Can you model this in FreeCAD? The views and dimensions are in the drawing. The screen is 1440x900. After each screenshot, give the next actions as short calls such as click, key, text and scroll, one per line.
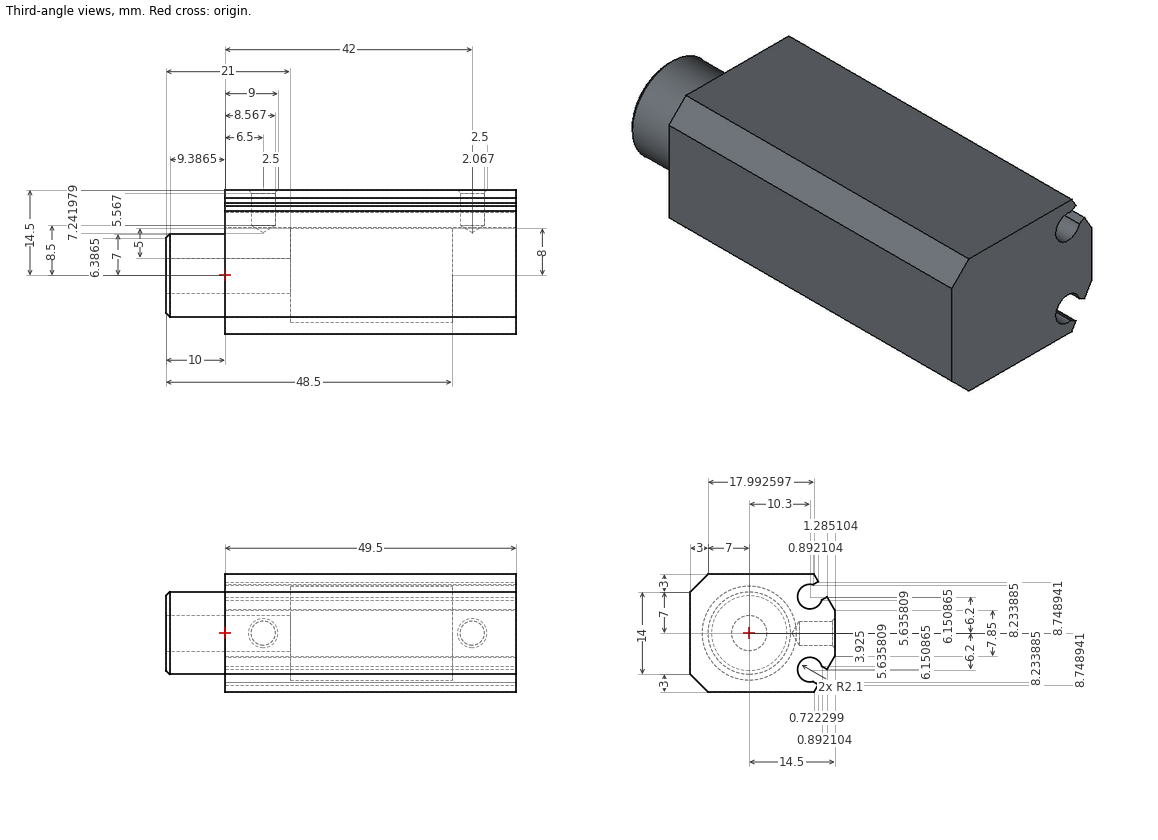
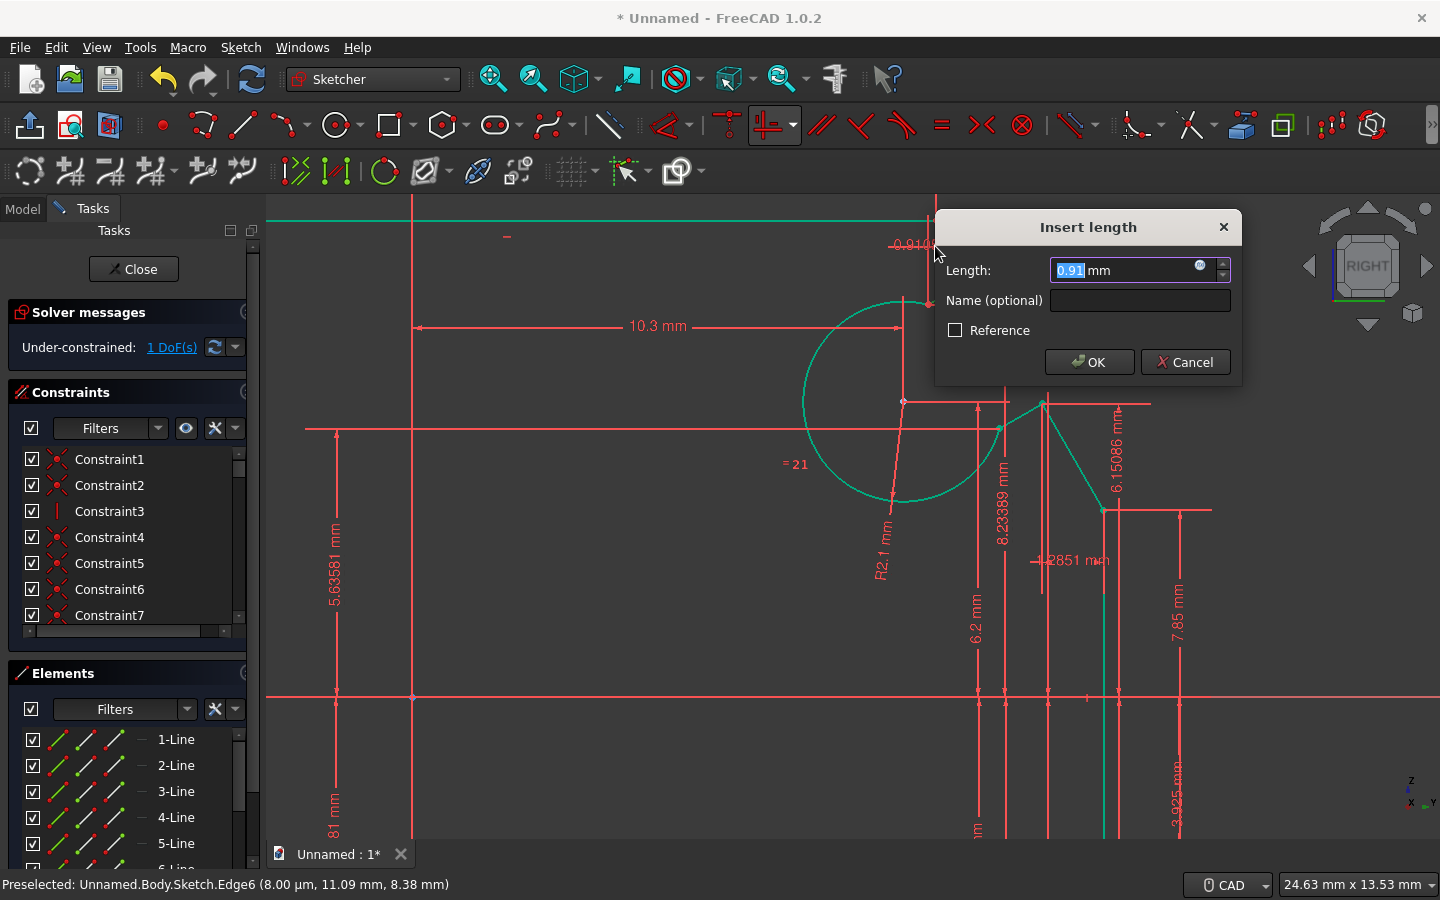
text(0.892104)
key(Return)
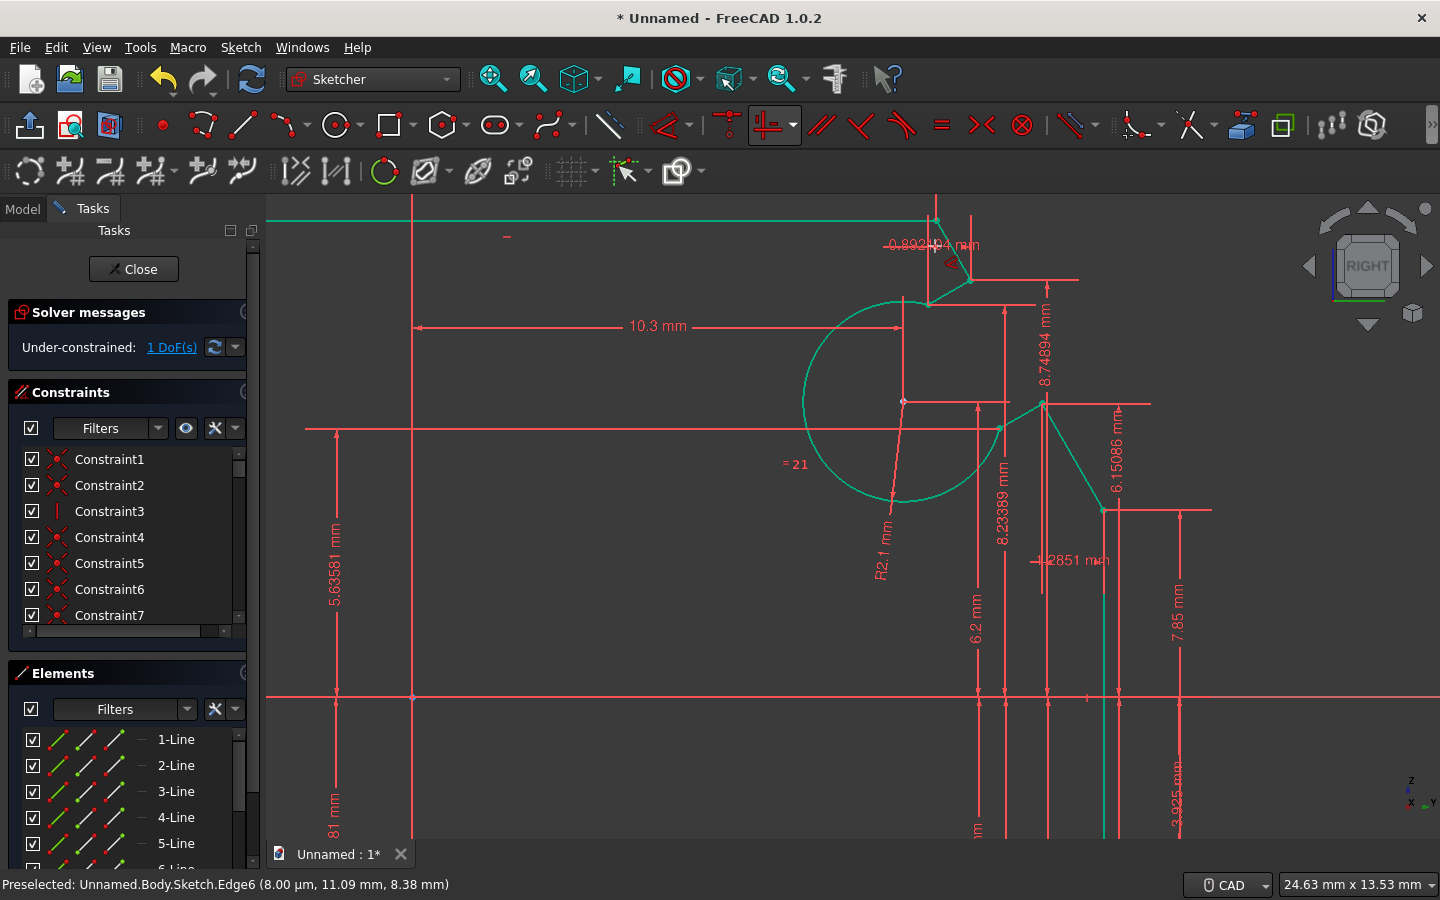
scroll(1001, 369, down, 4)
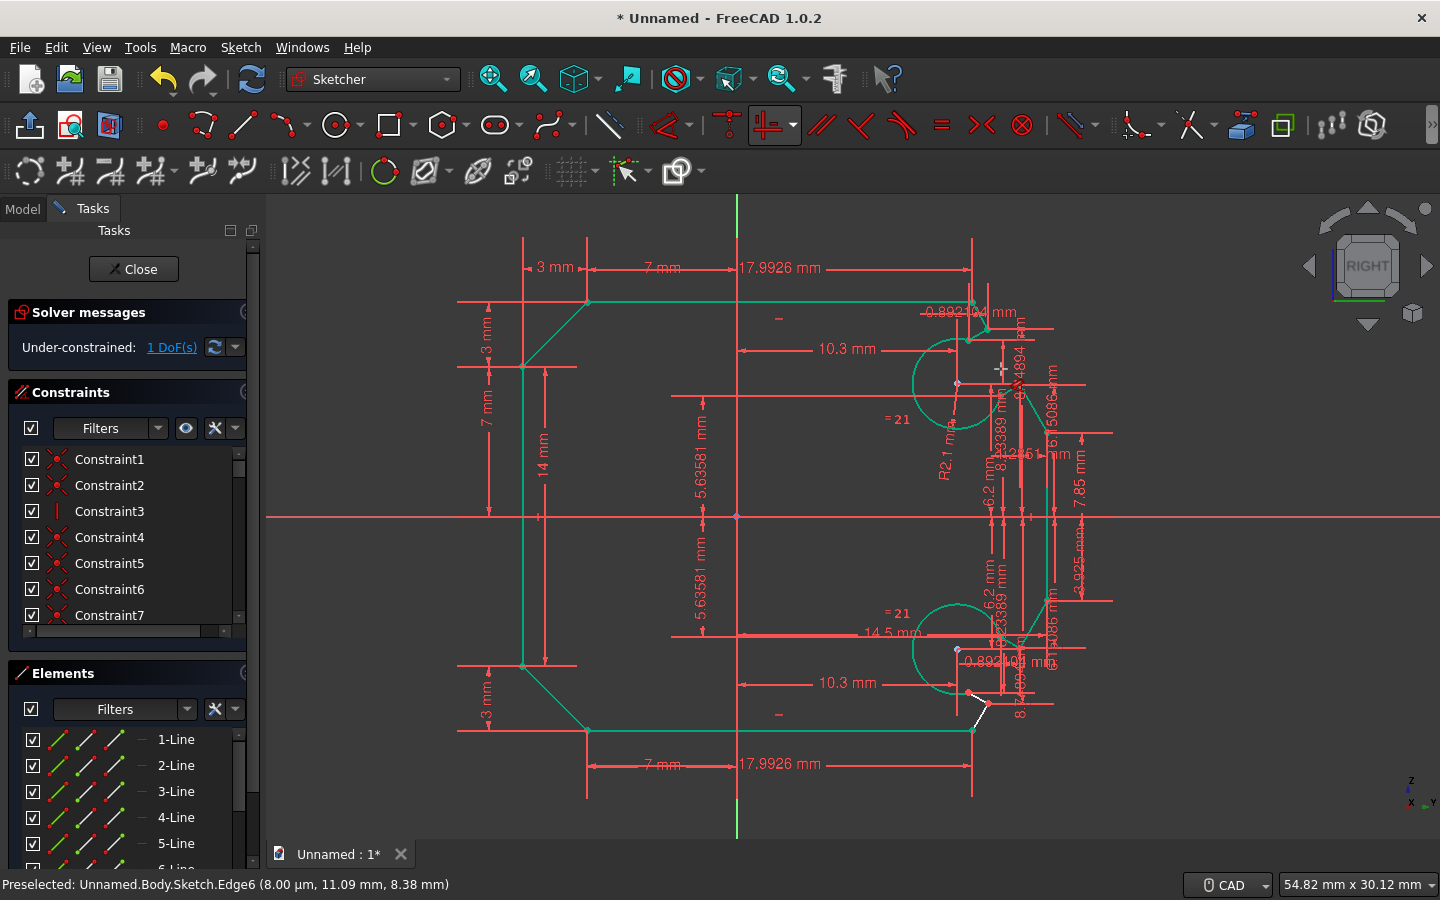
scroll(977, 723, up, 5)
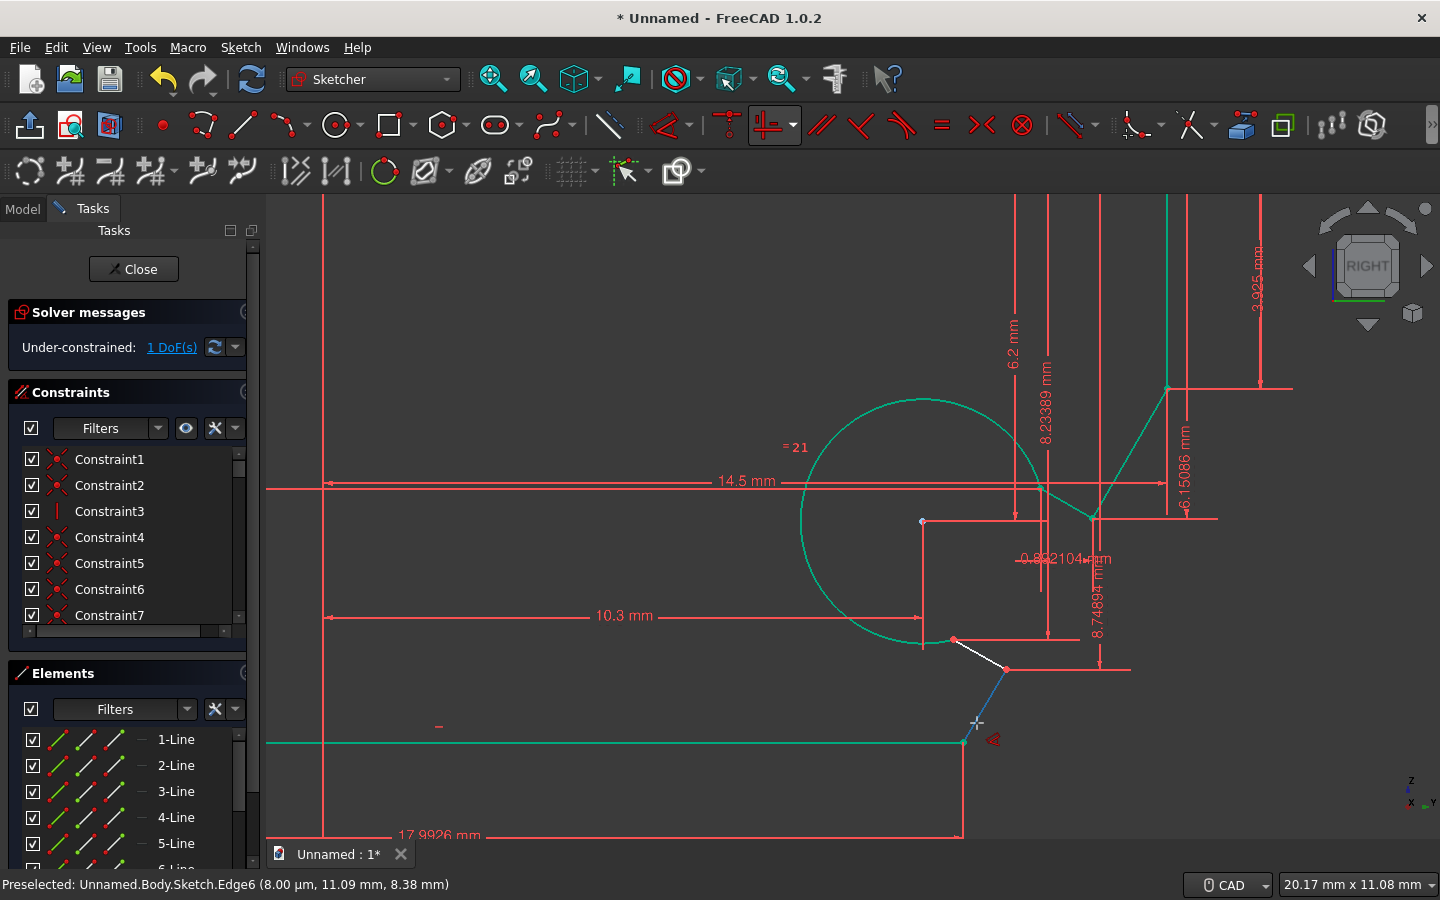
click(976, 721)
click(985, 777)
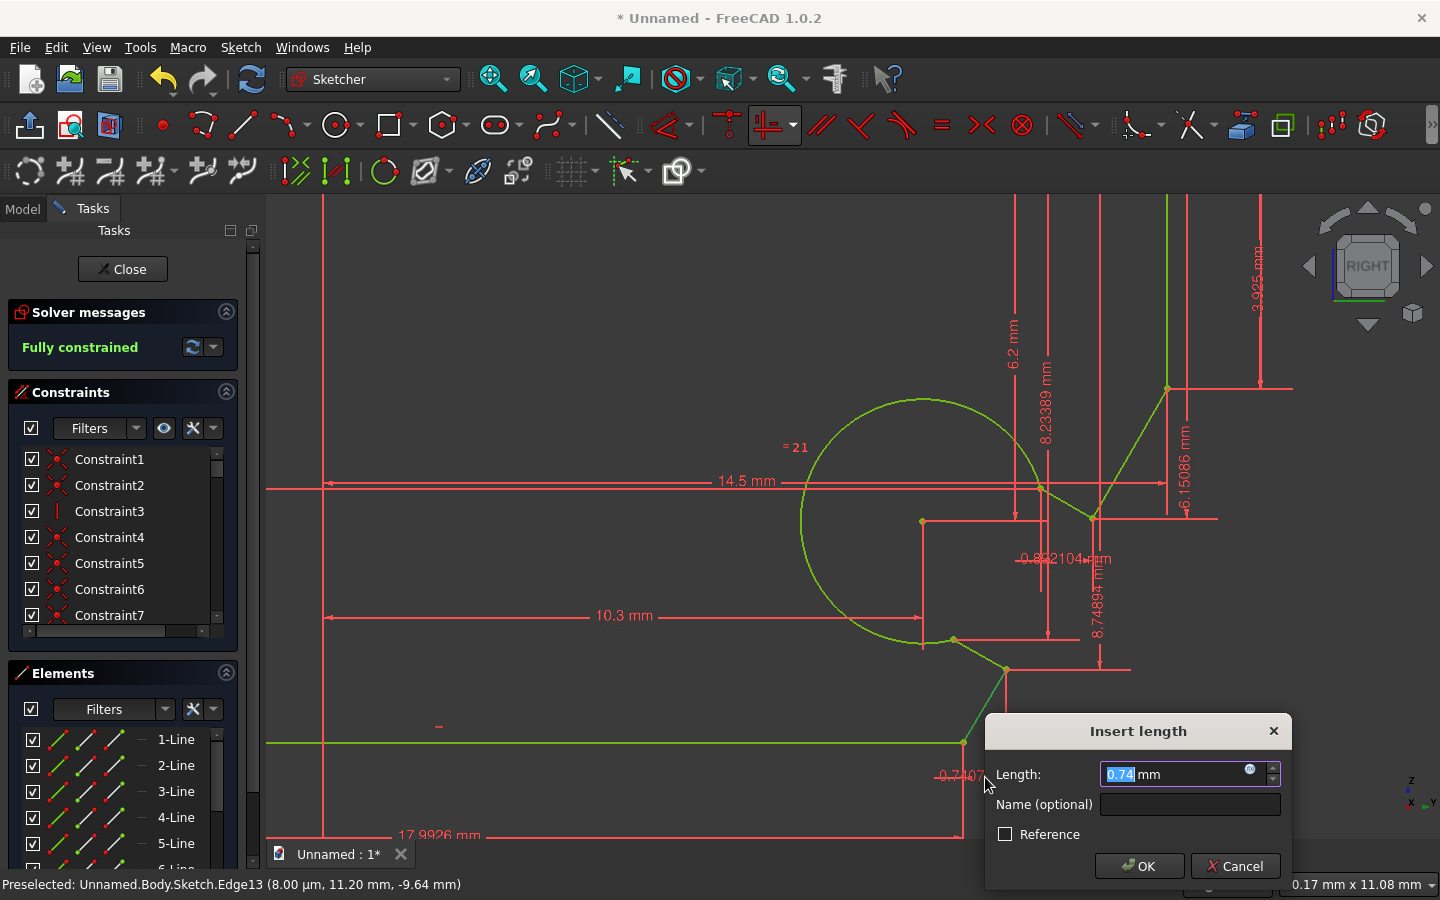
text(0.722299)
key(Return)
key(Escape)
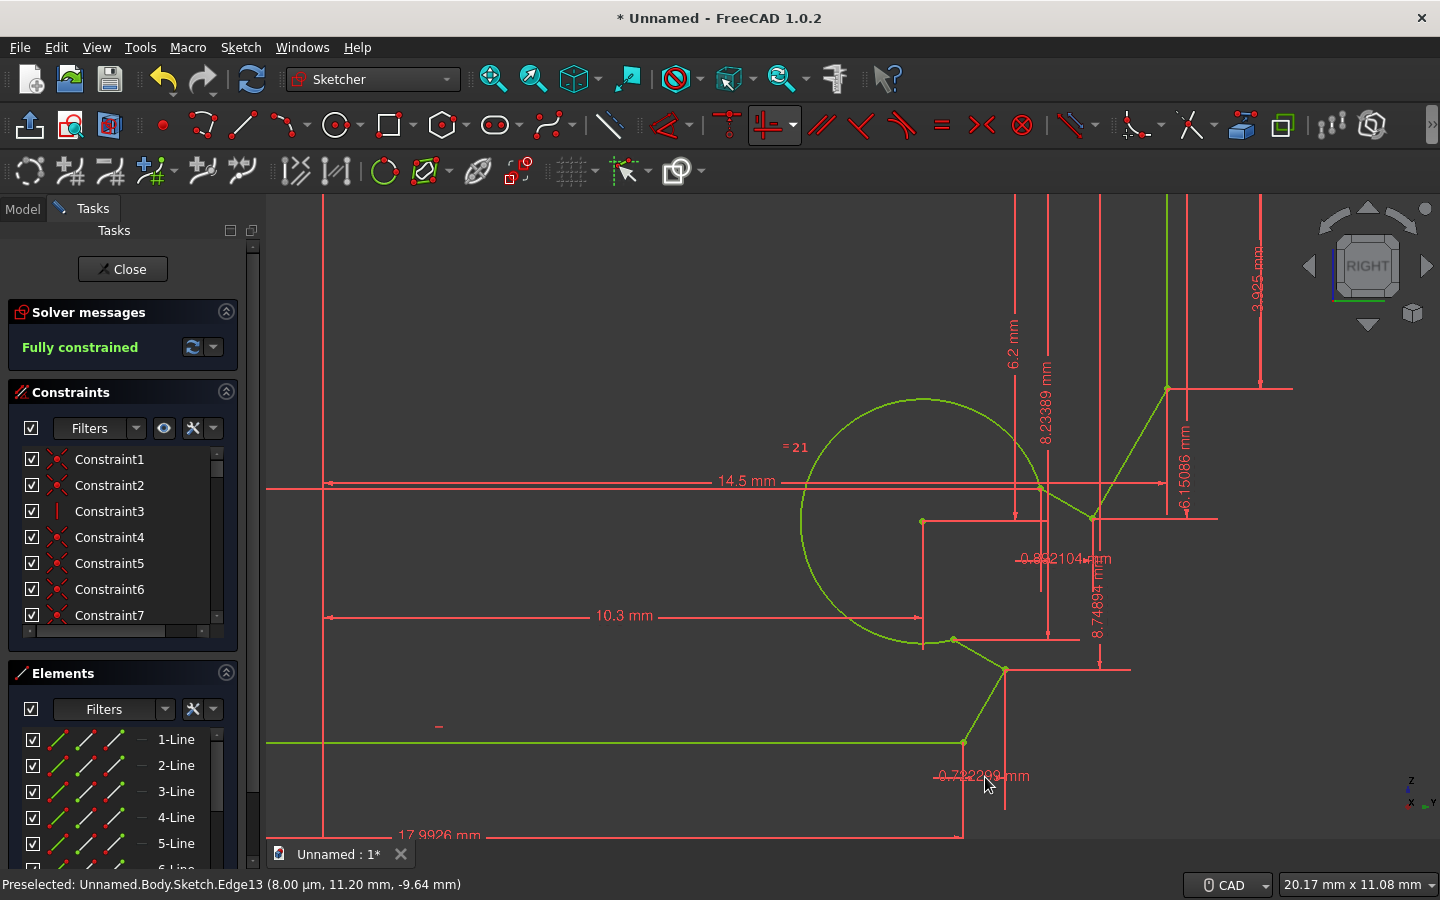
click(123, 269)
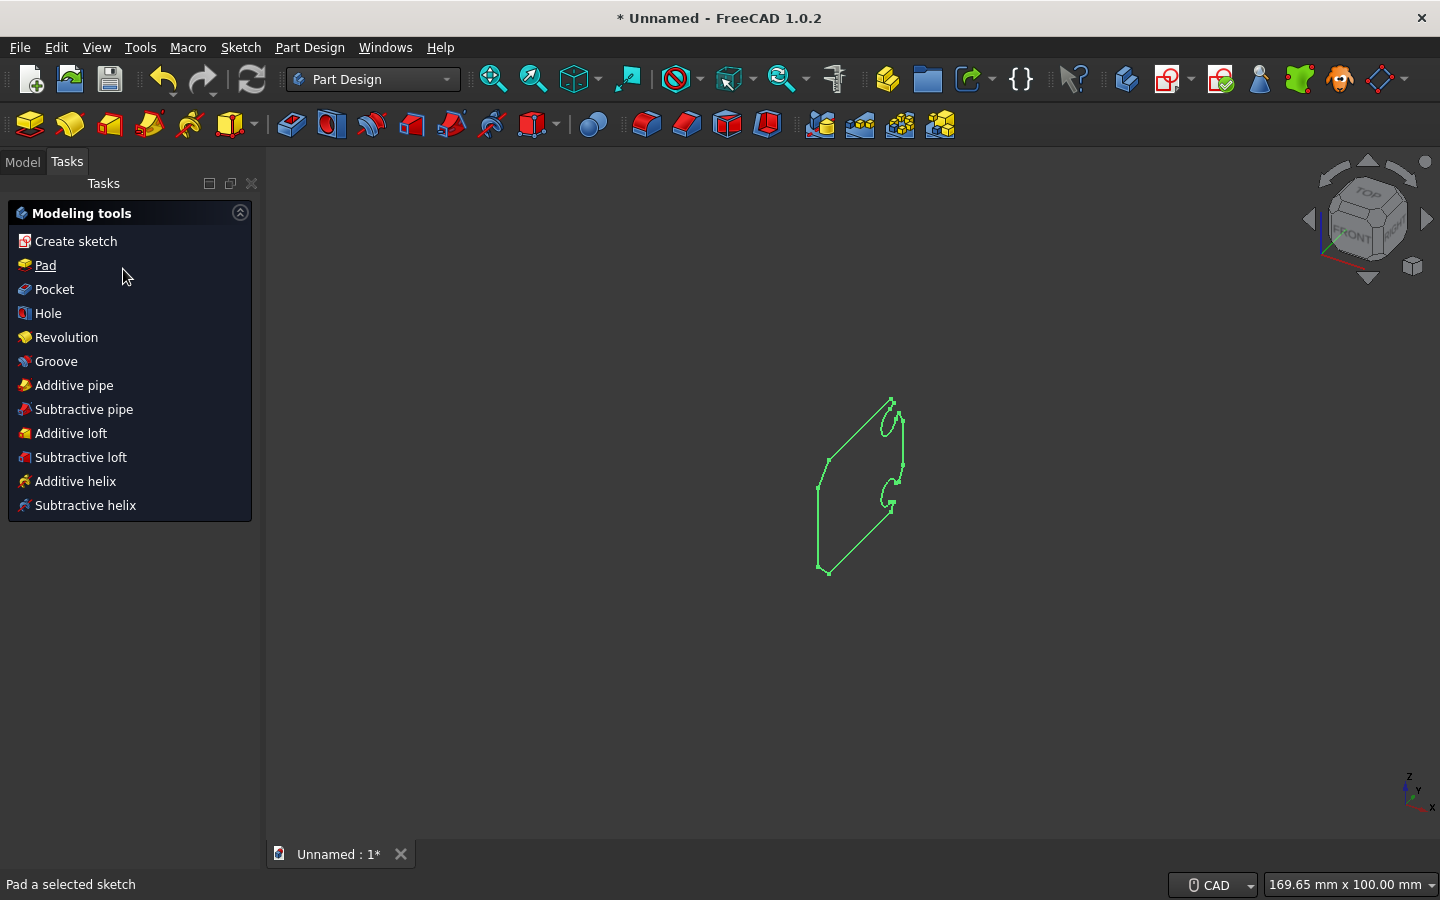
click(30, 124)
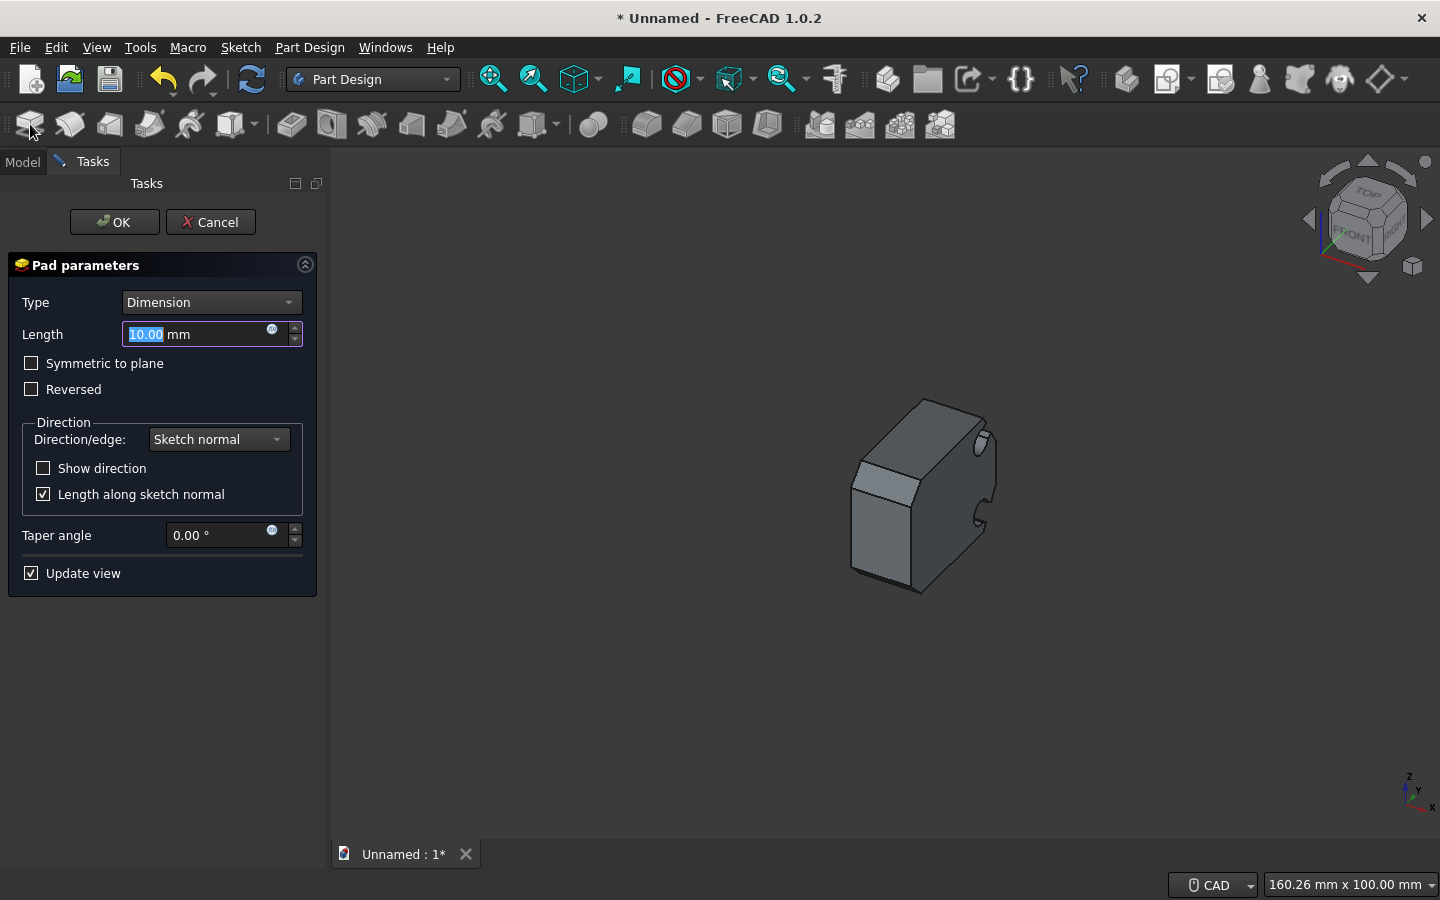
text(49.5)
key(Tab)